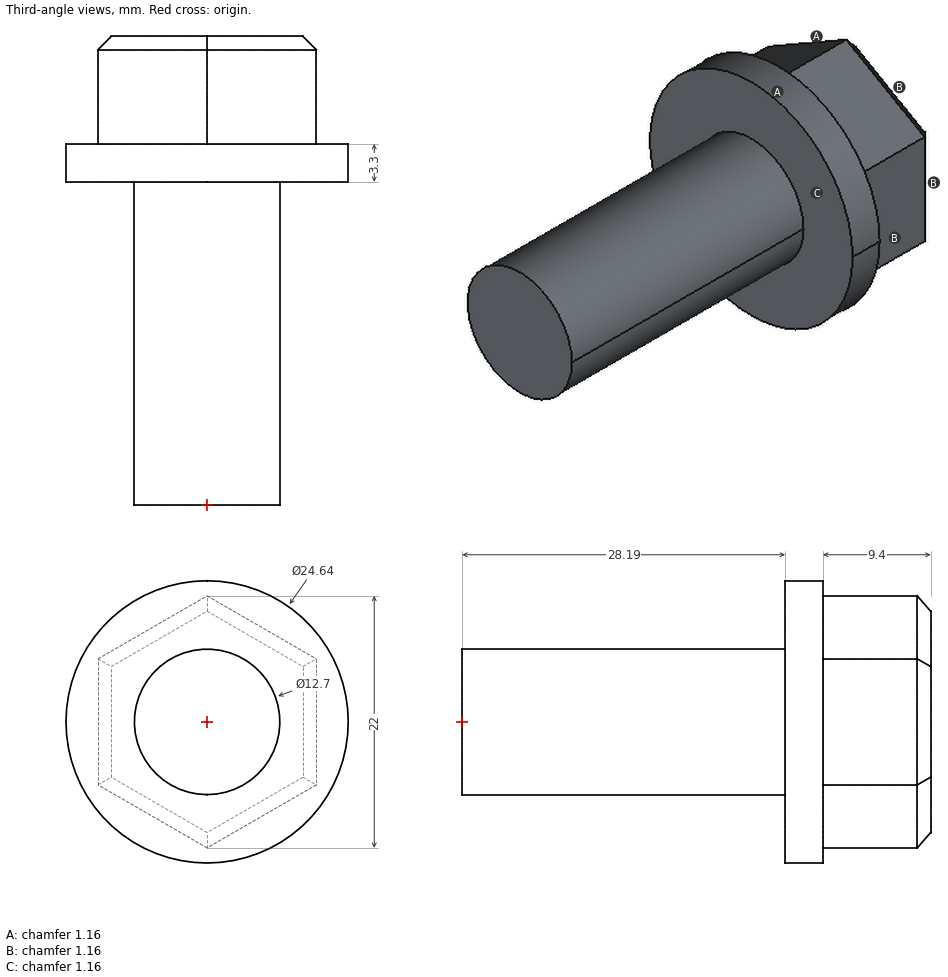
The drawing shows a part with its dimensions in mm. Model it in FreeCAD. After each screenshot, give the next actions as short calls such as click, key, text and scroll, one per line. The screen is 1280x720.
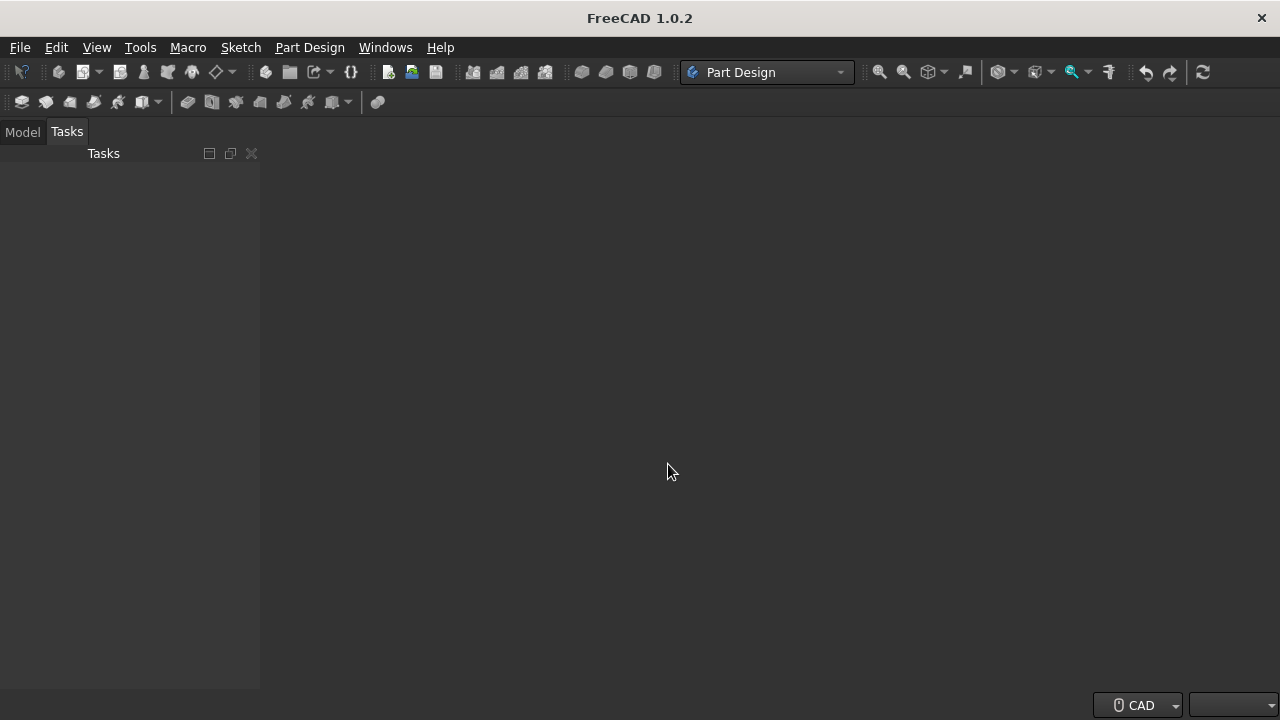
click(388, 72)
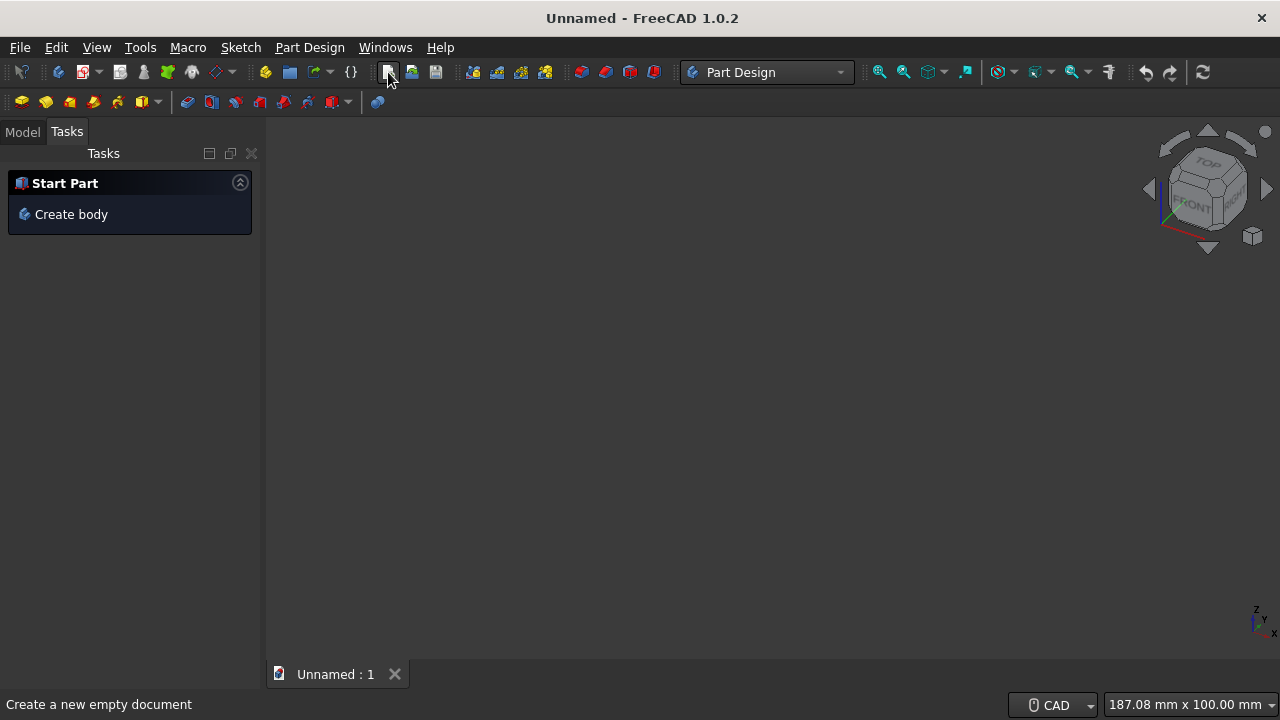
click(84, 72)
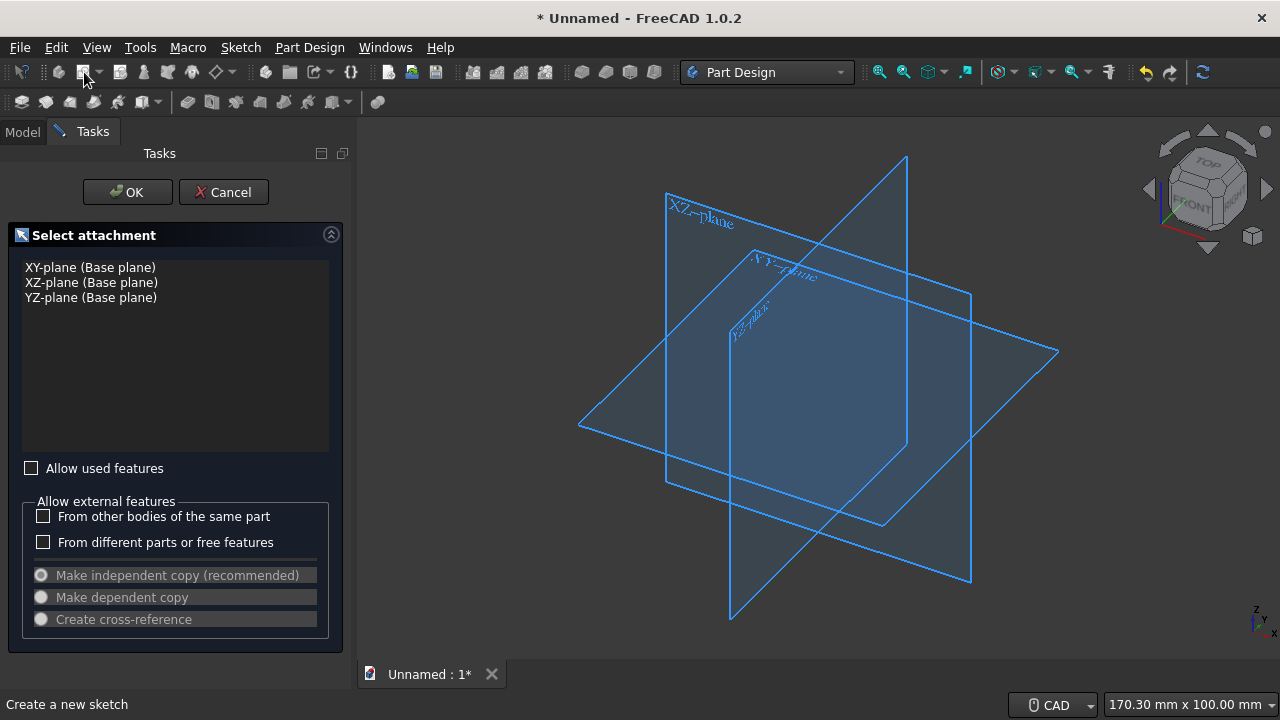
click(82, 282)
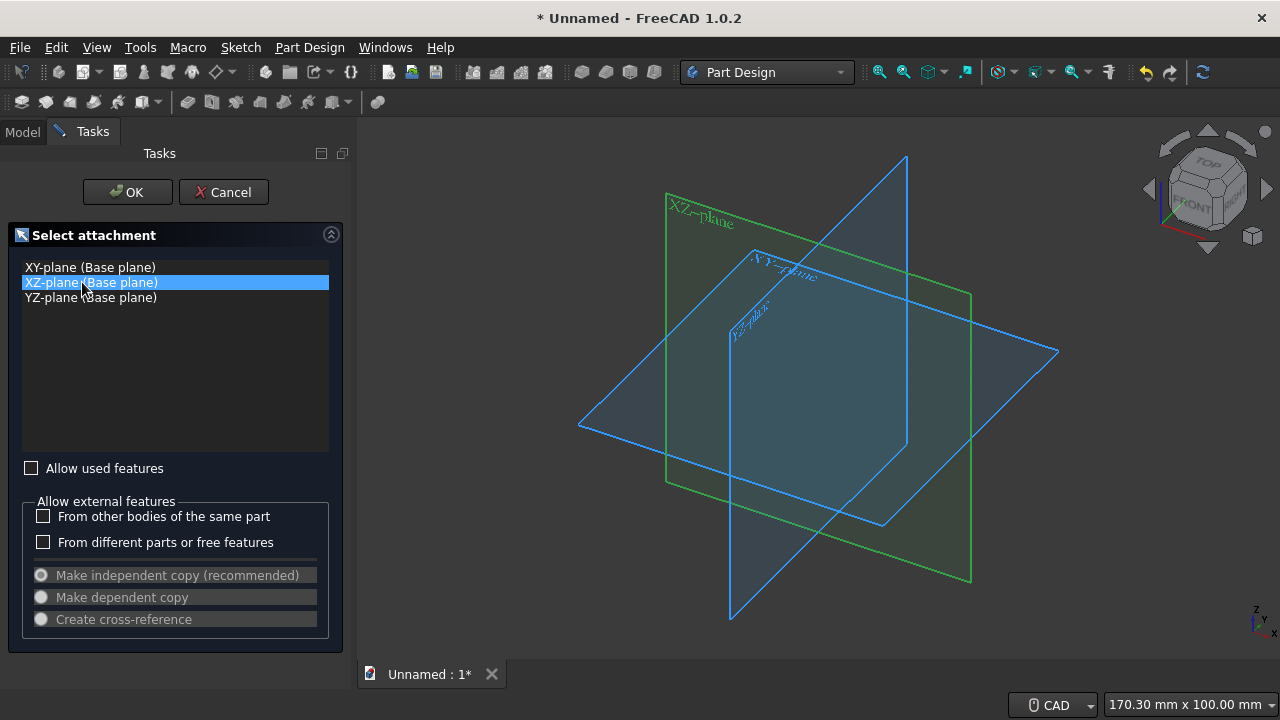
click(128, 192)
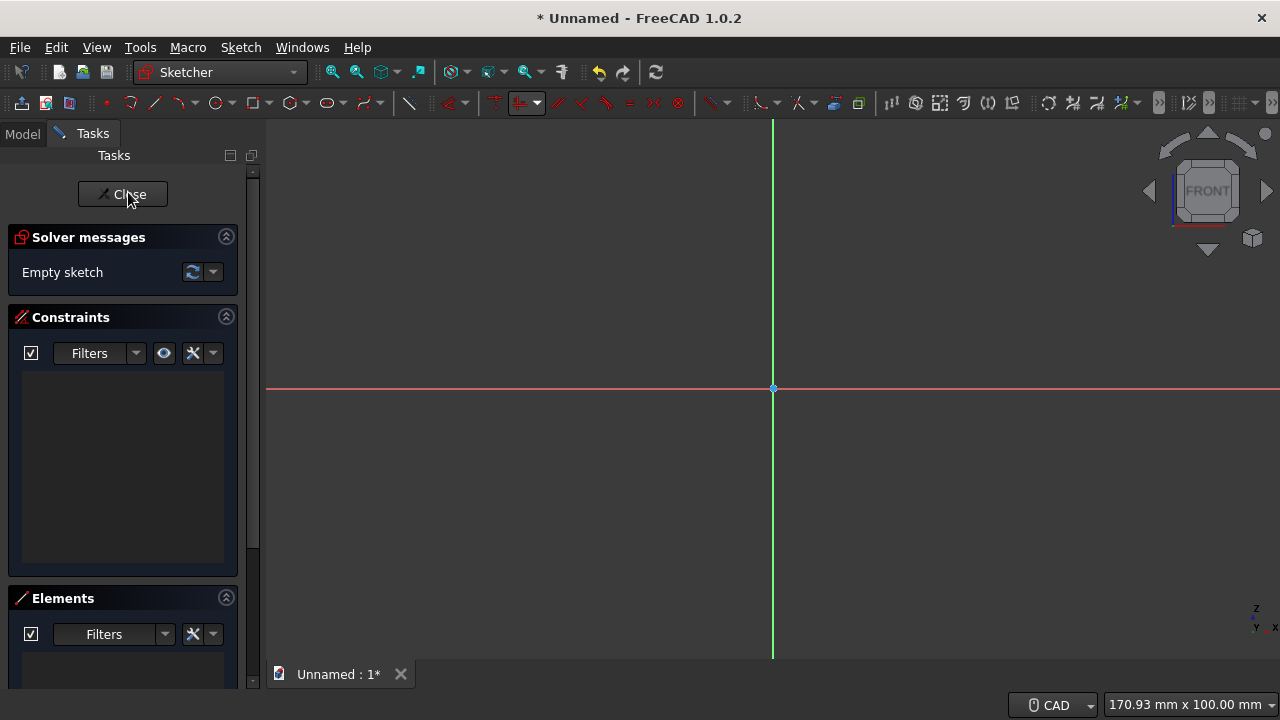
scroll(790, 389, up, 8)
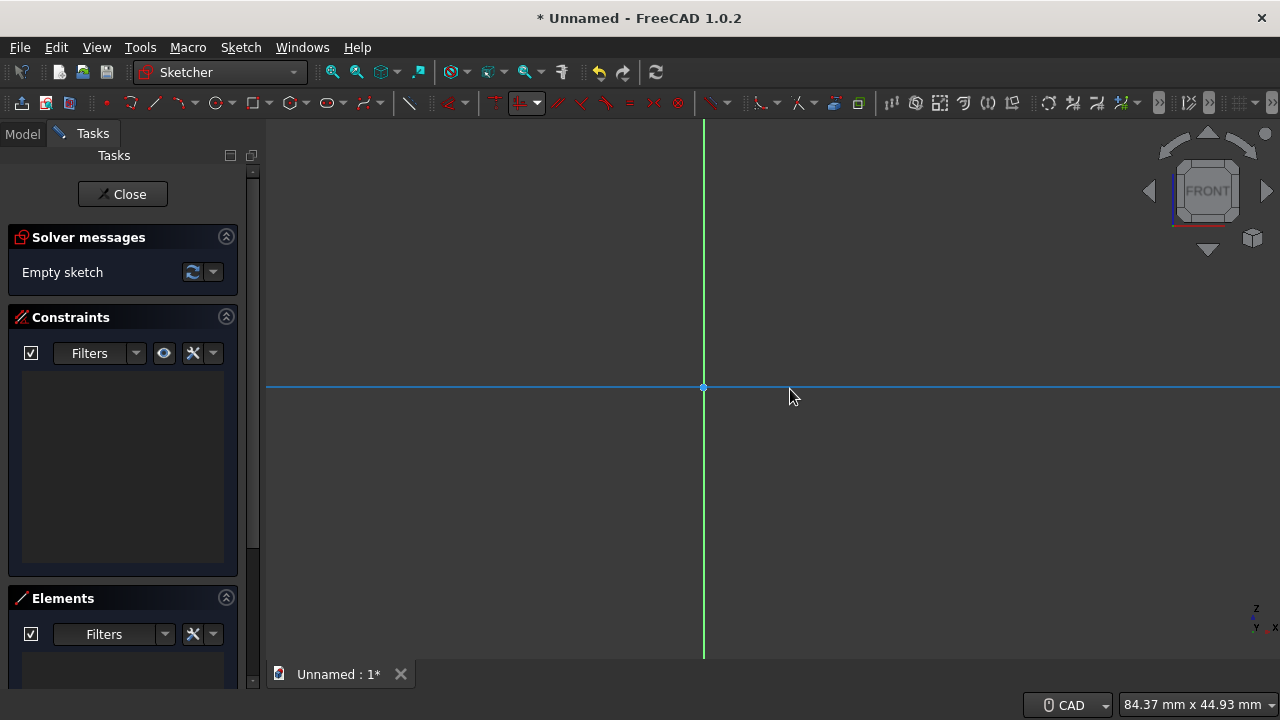
click(216, 104)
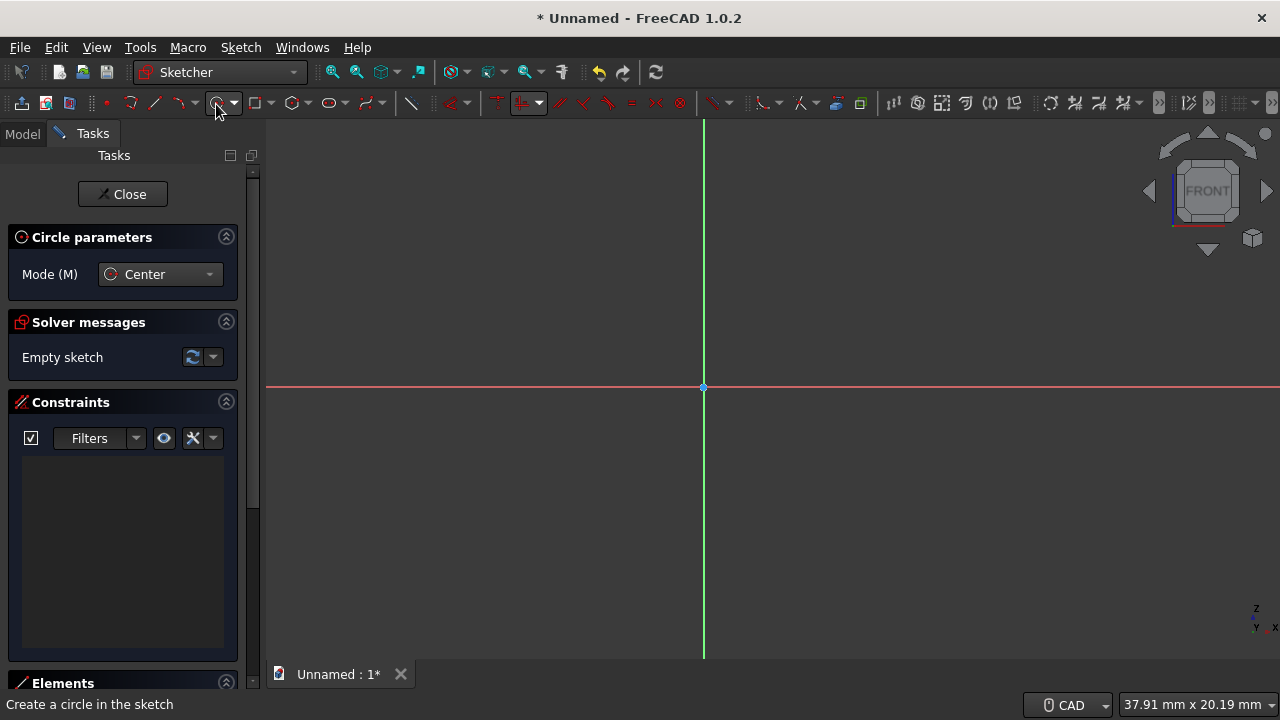
click(704, 387)
move(824, 267)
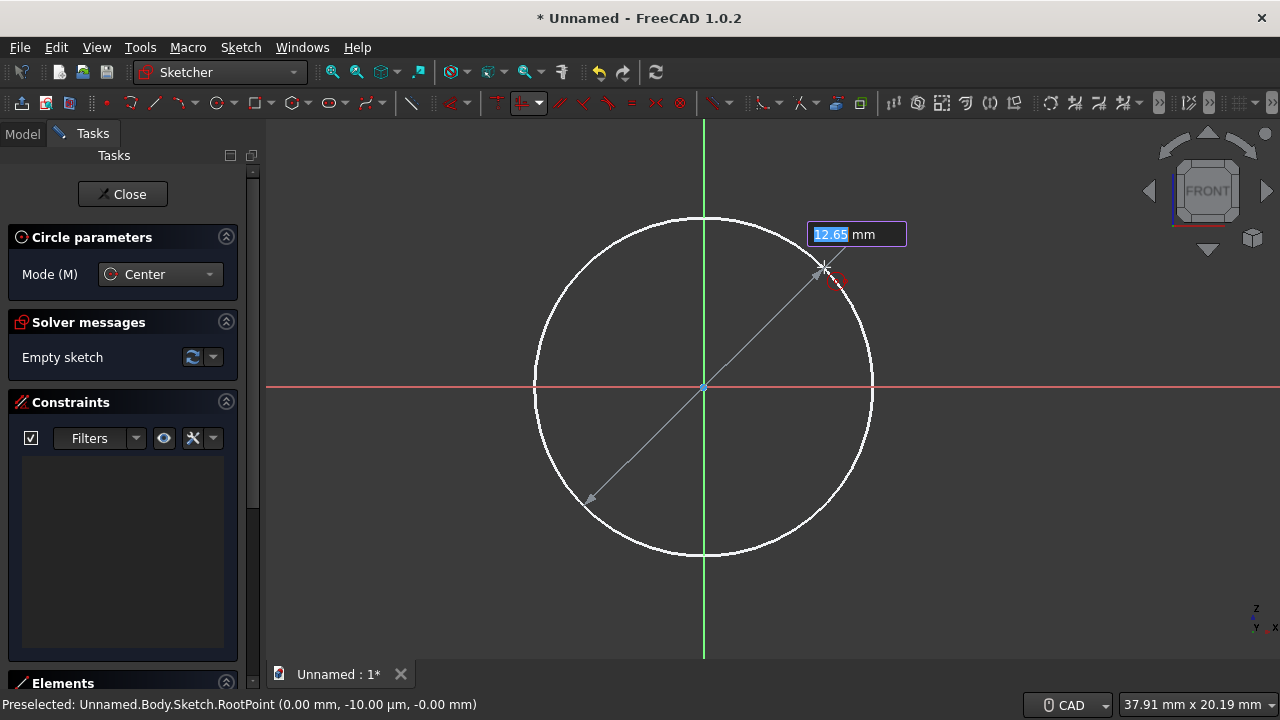
text(12.7)
key(Return)
key(Escape)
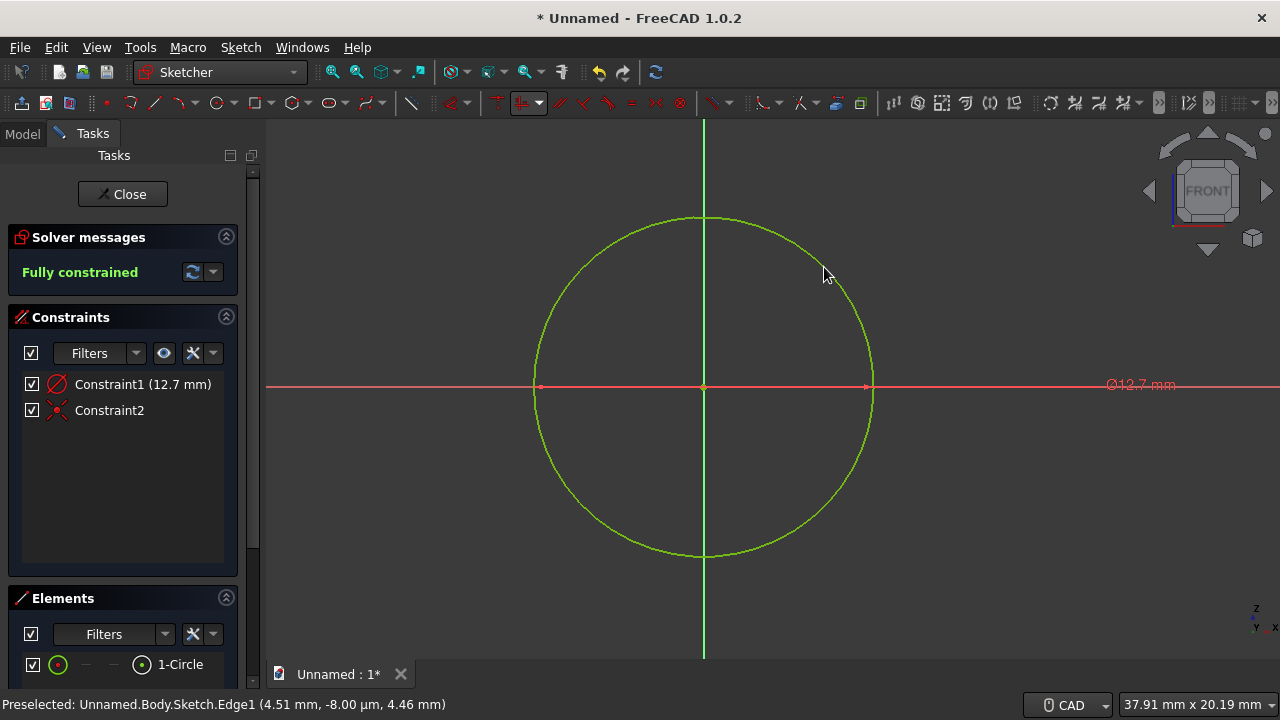
click(123, 194)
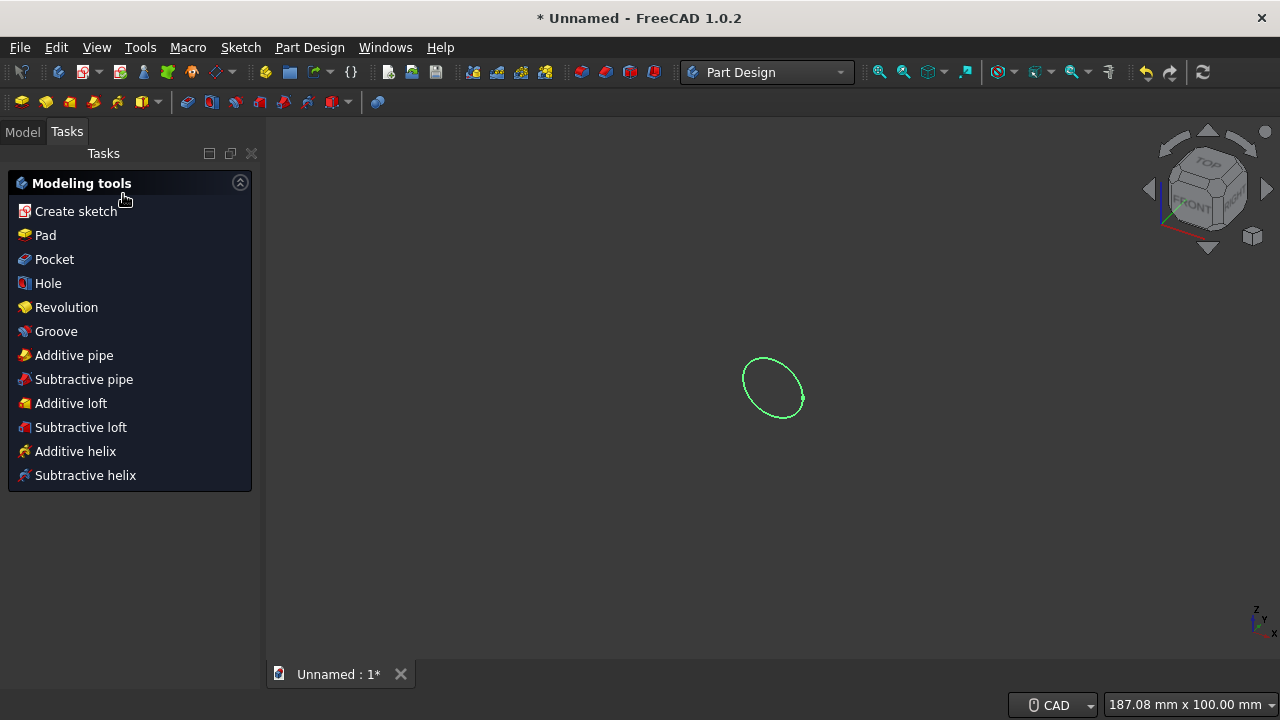
click(22, 102)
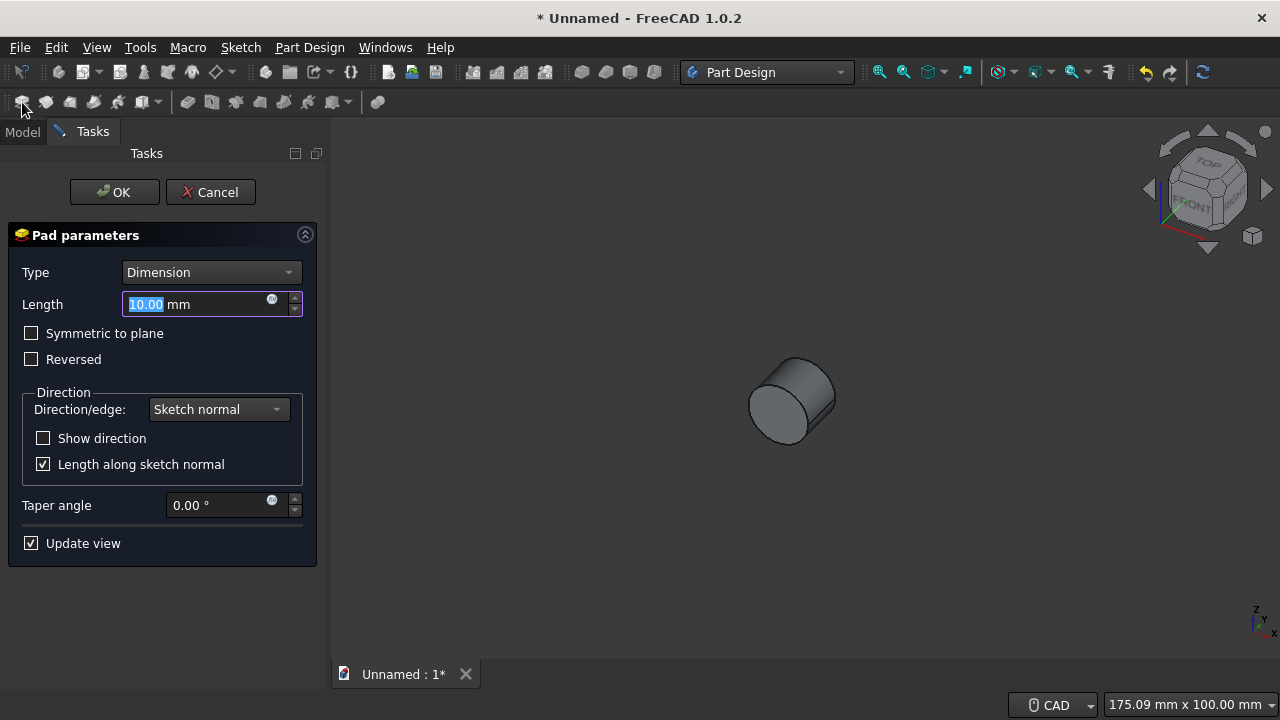
text(28.19)
key(Tab)